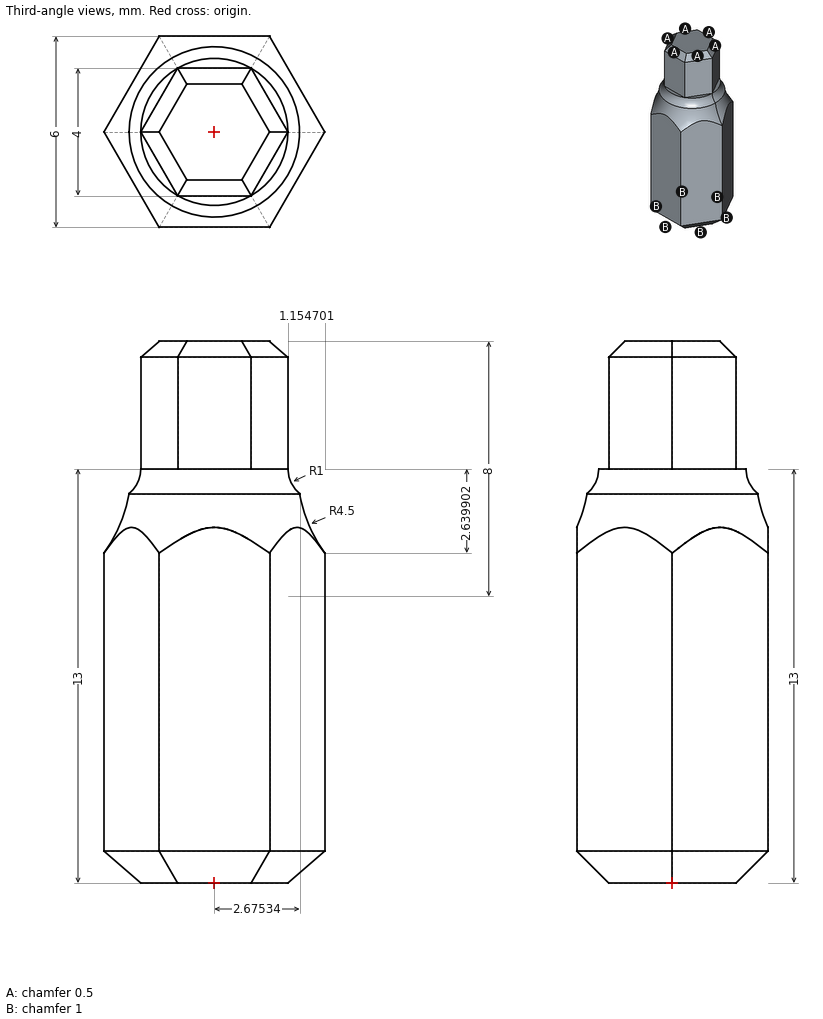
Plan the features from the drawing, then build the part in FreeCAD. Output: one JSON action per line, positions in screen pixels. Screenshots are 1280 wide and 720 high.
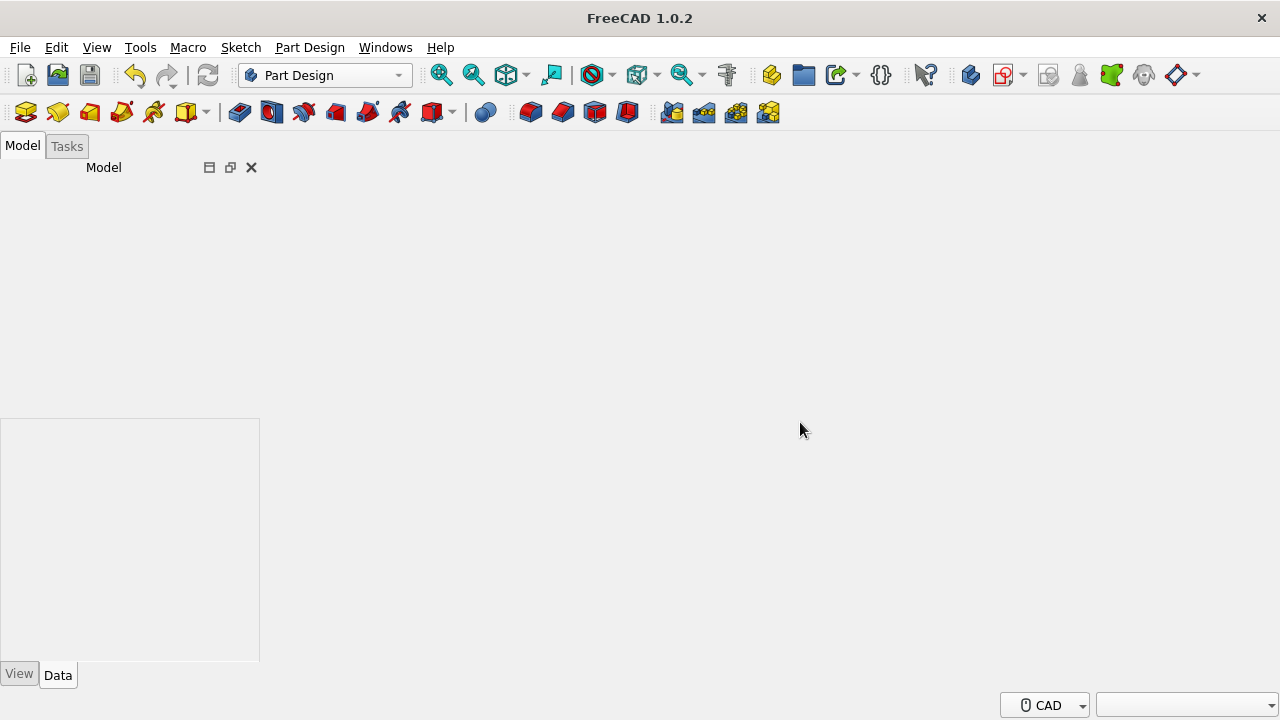
{"action": "left_click", "coordinate": [26, 76]}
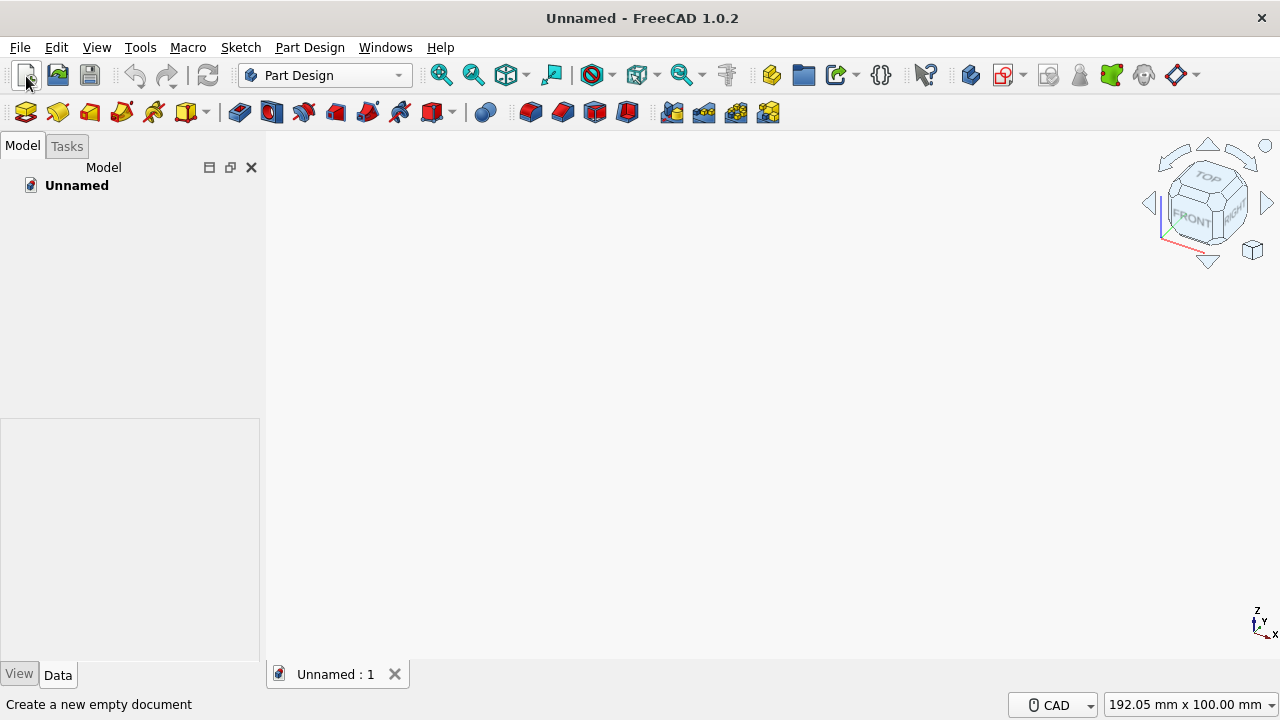
{"action": "left_click", "coordinate": [1004, 76]}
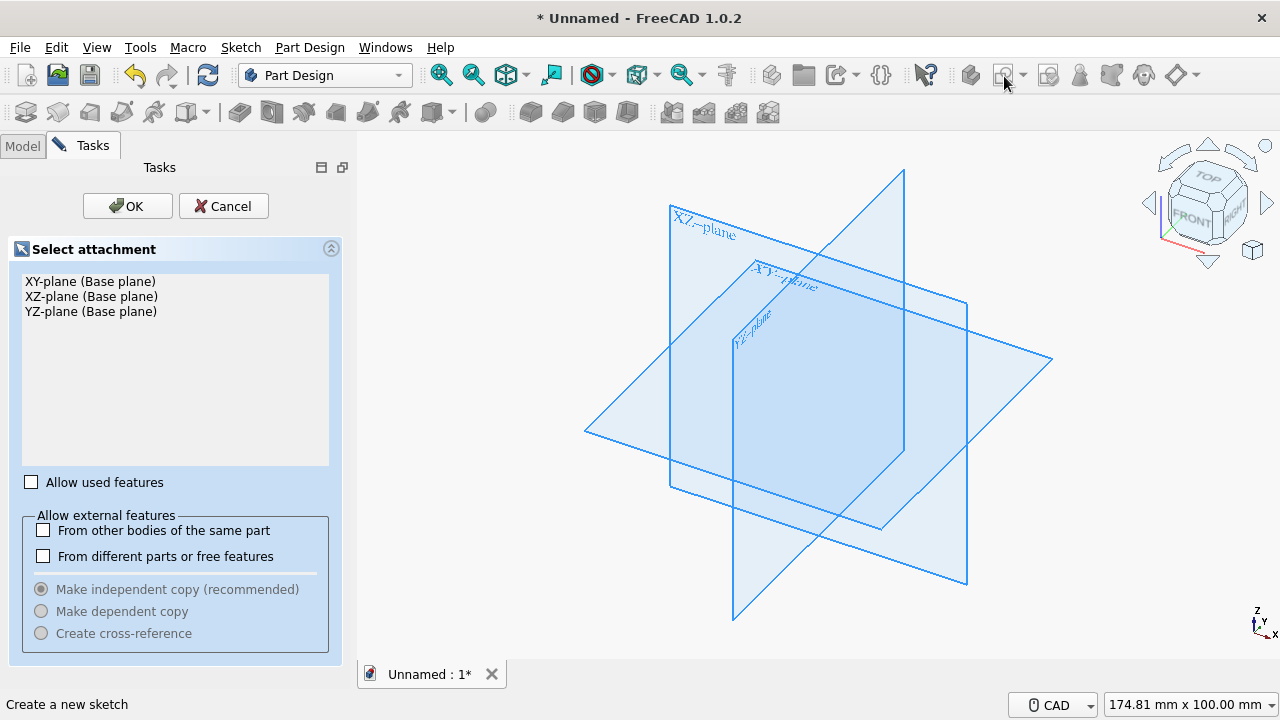
{"action": "left_click", "coordinate": [82, 282]}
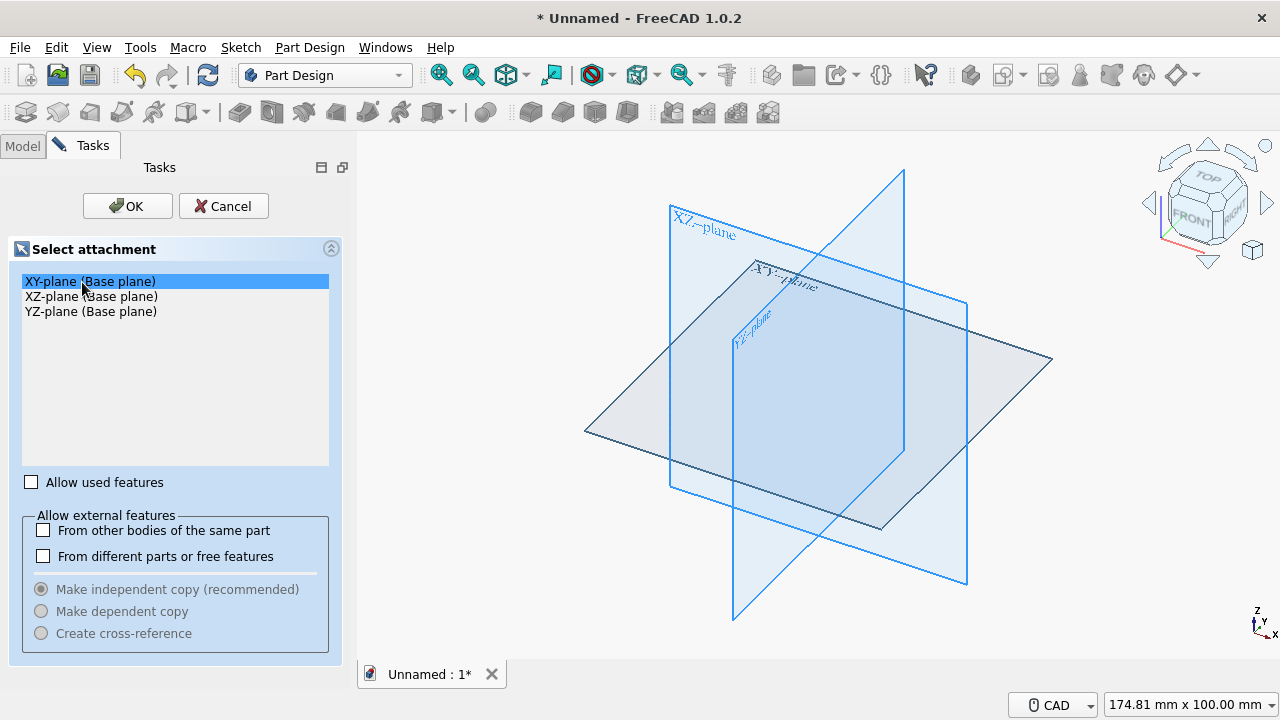
{"action": "left_click", "coordinate": [128, 206]}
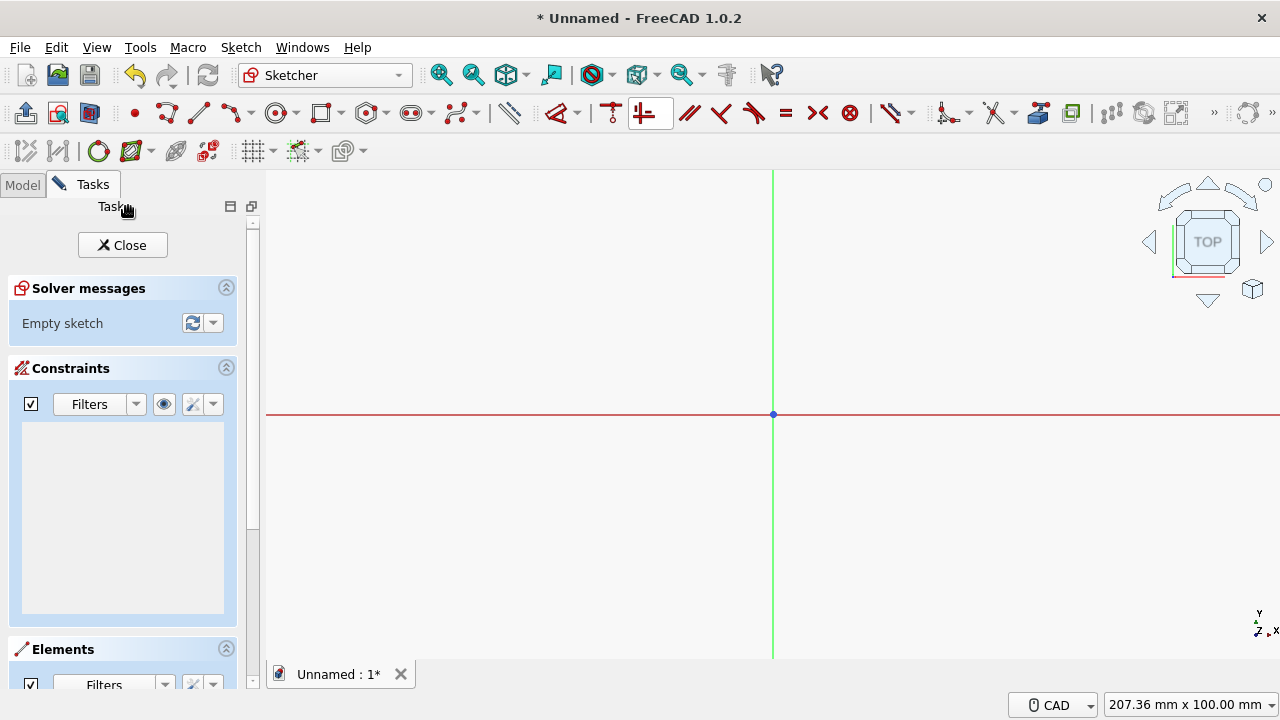
{"action": "scroll", "coordinate": [780, 414], "scroll_direction": "up", "scroll_amount": 12}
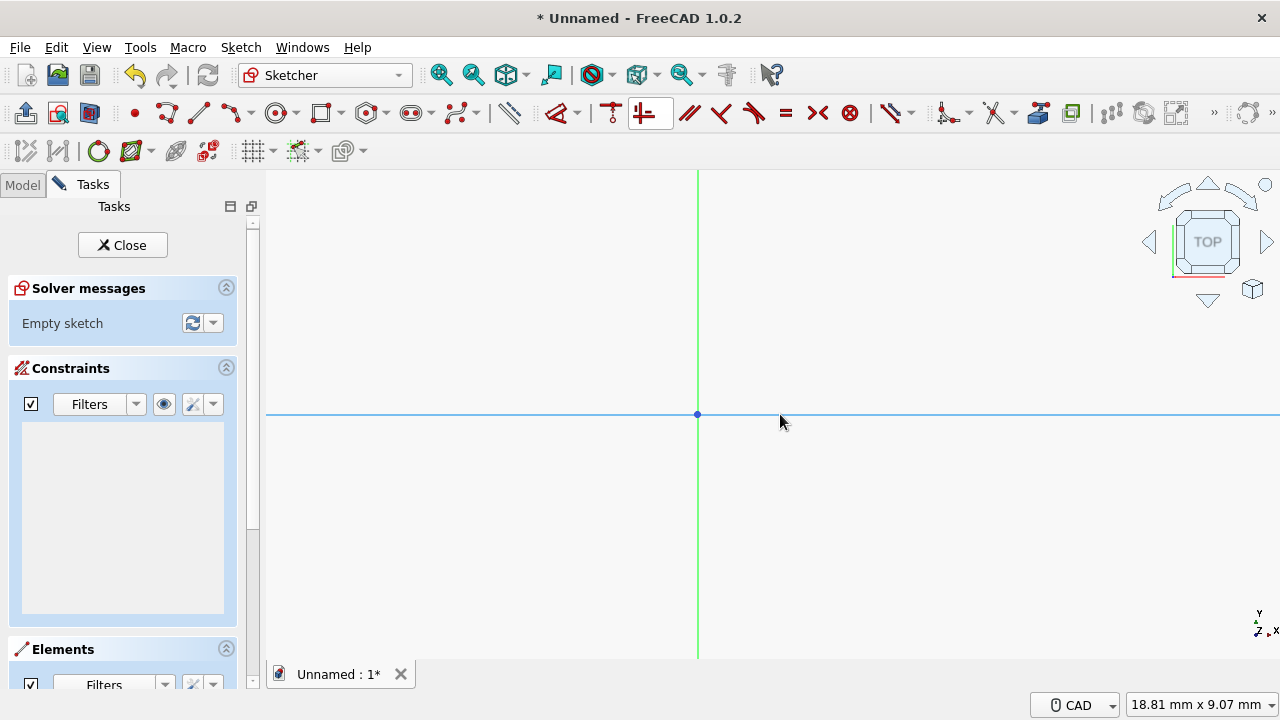
{"action": "left_click", "coordinate": [366, 114]}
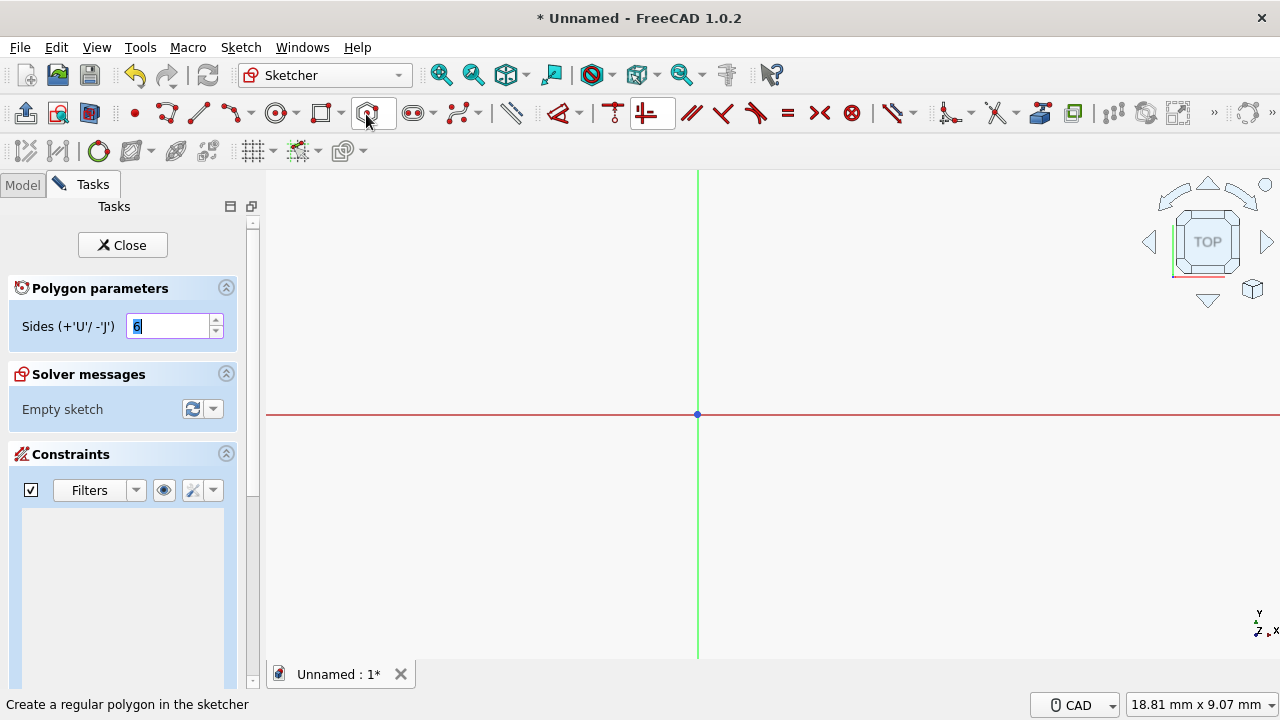
{"action": "left_click", "coordinate": [698, 414]}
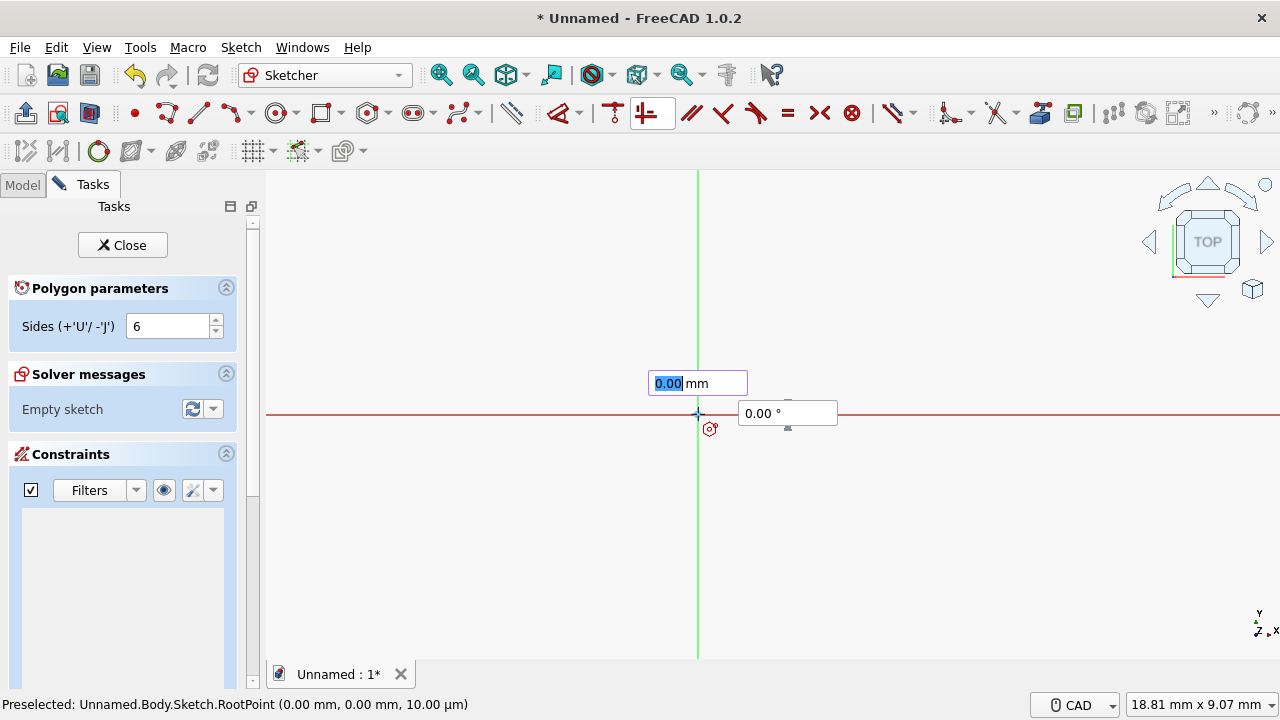
{"action": "left_click", "coordinate": [884, 414]}
{"action": "right_click", "coordinate": [884, 414]}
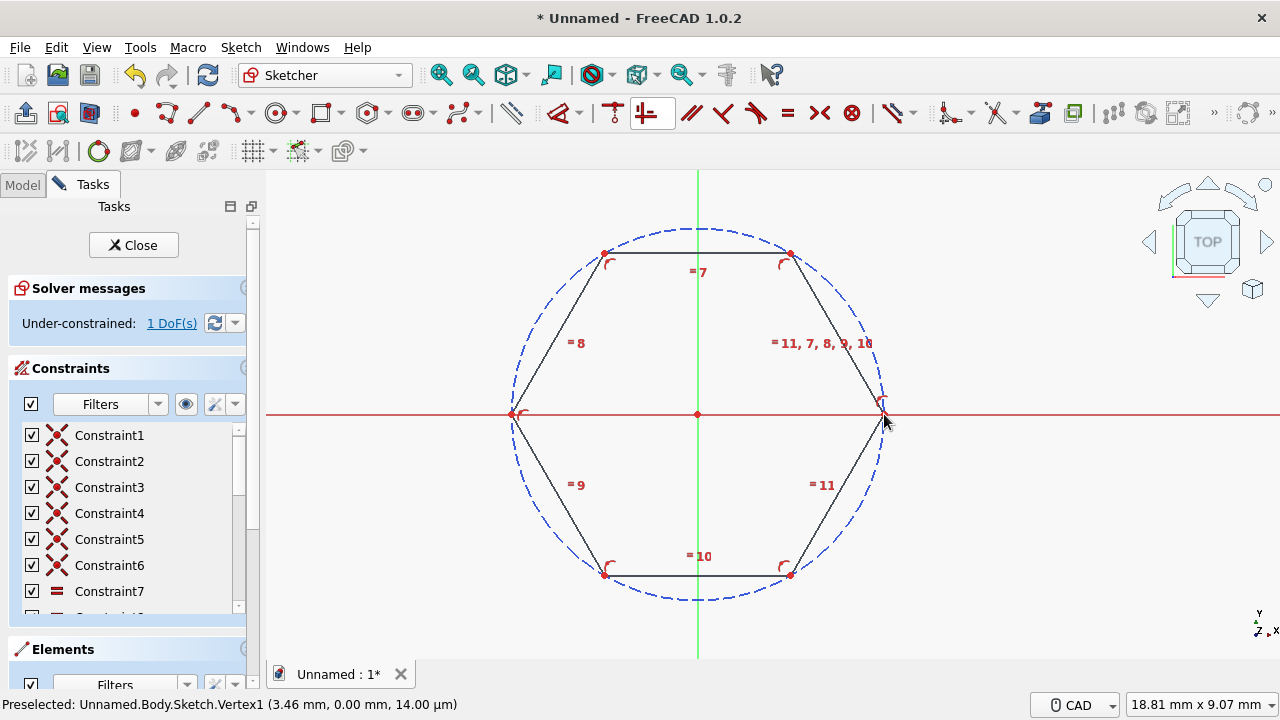
{"action": "left_click", "coordinate": [558, 114]}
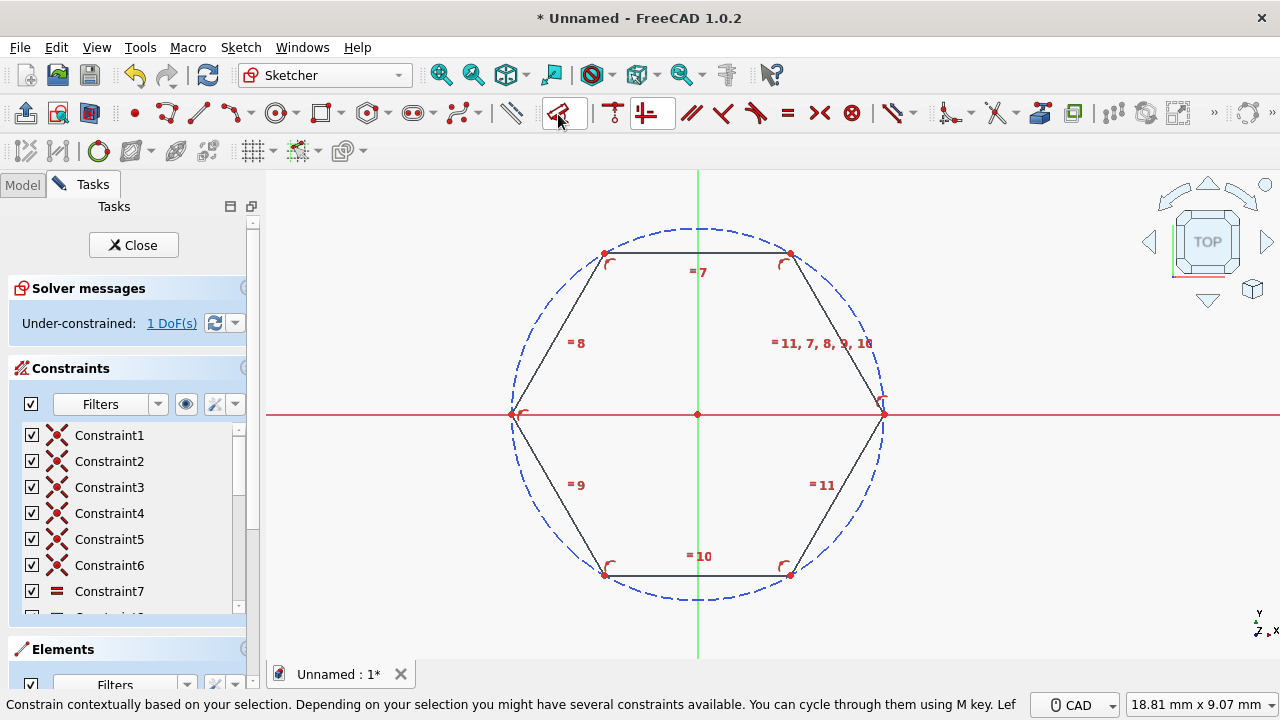
{"action": "left_click", "coordinate": [605, 576]}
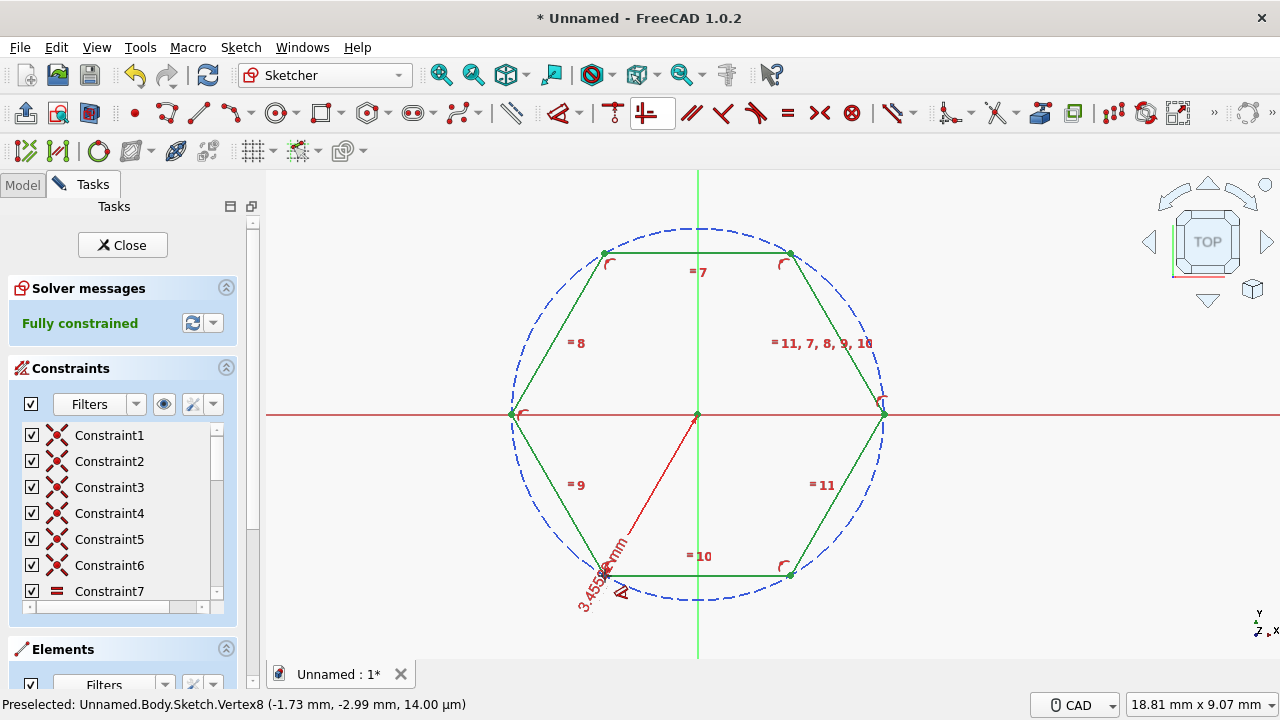
{"action": "left_click", "coordinate": [791, 253]}
{"action": "left_click", "coordinate": [825, 340]}